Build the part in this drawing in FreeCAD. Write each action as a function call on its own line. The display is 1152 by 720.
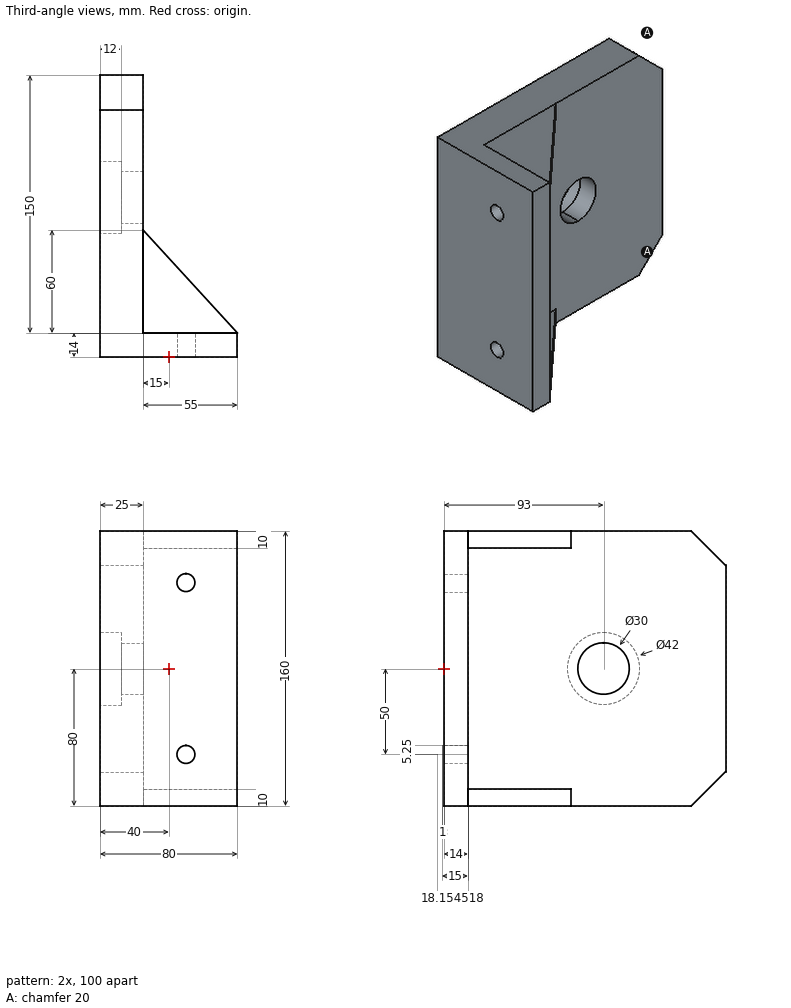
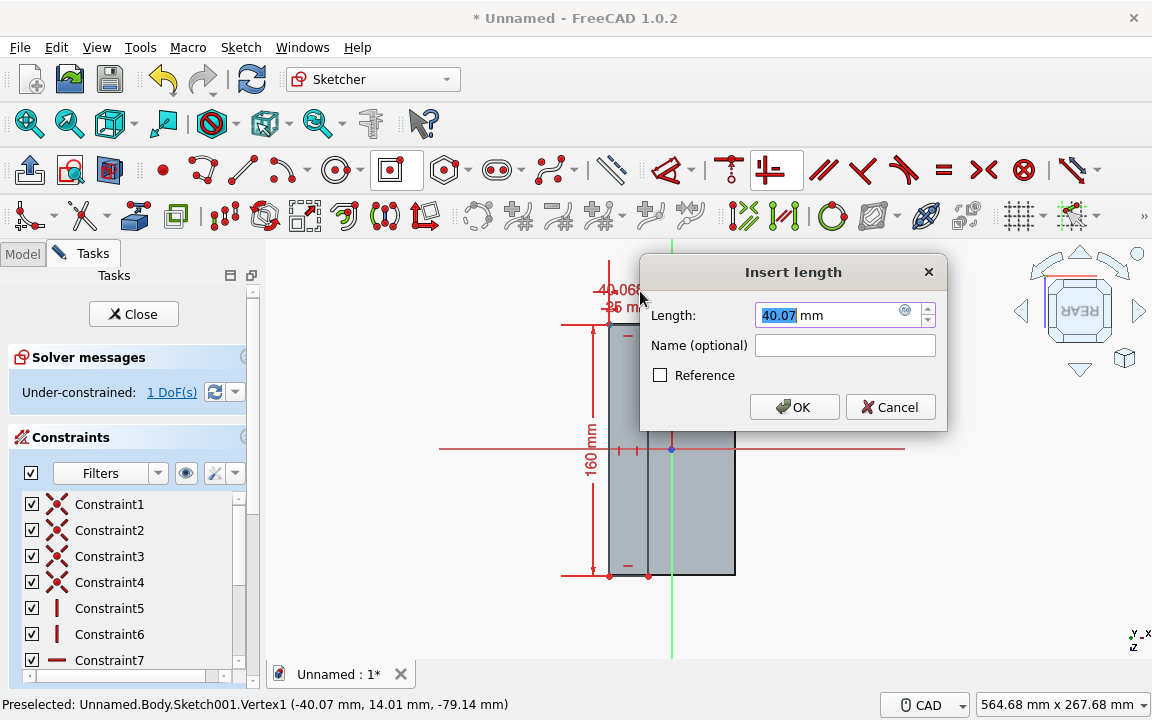
text(40)
key(Return)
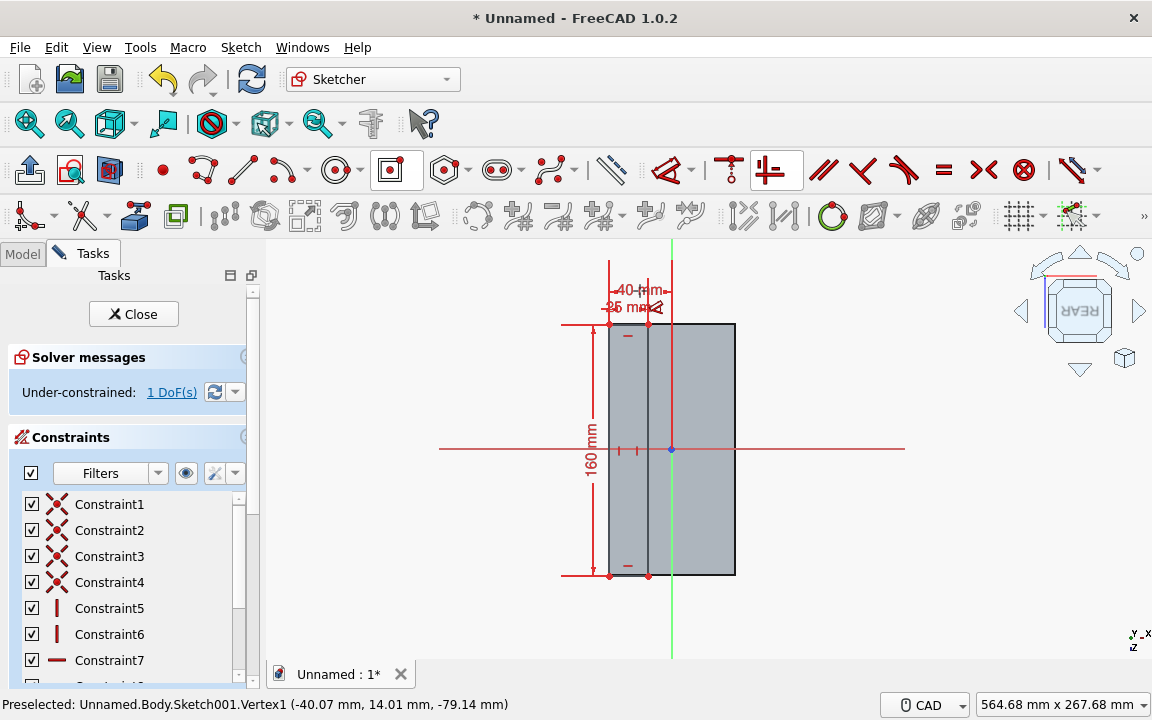
click(609, 325)
click(706, 387)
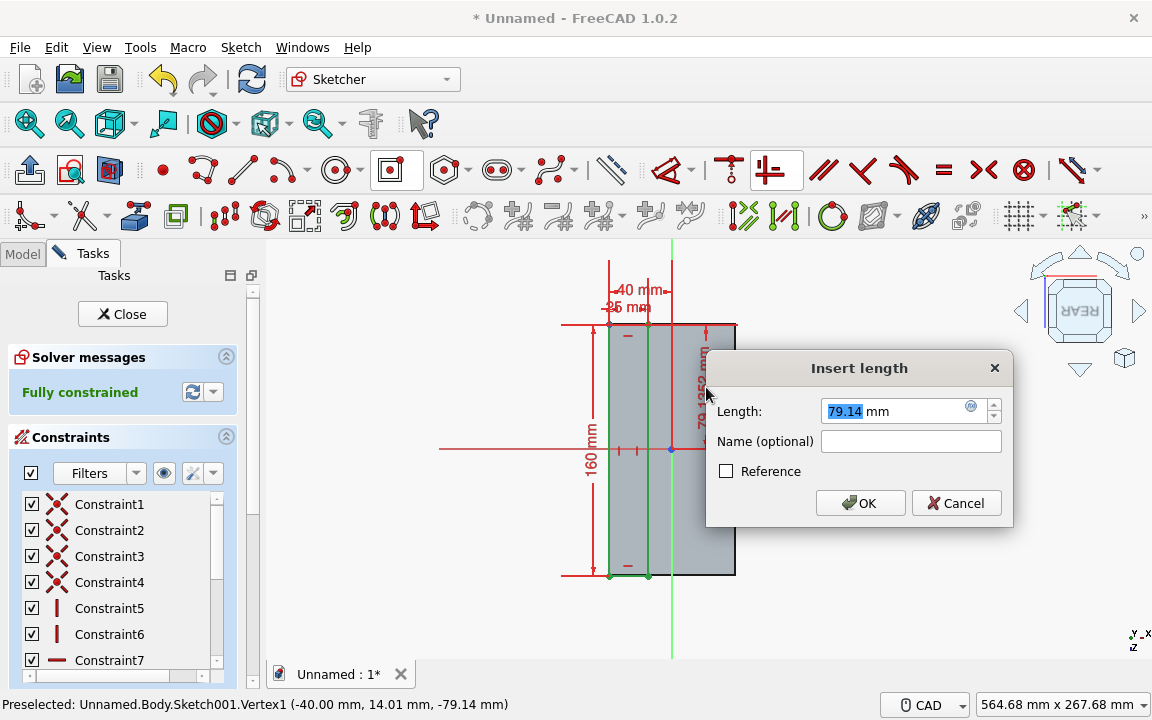
text(80)
key(Return)
key(Escape)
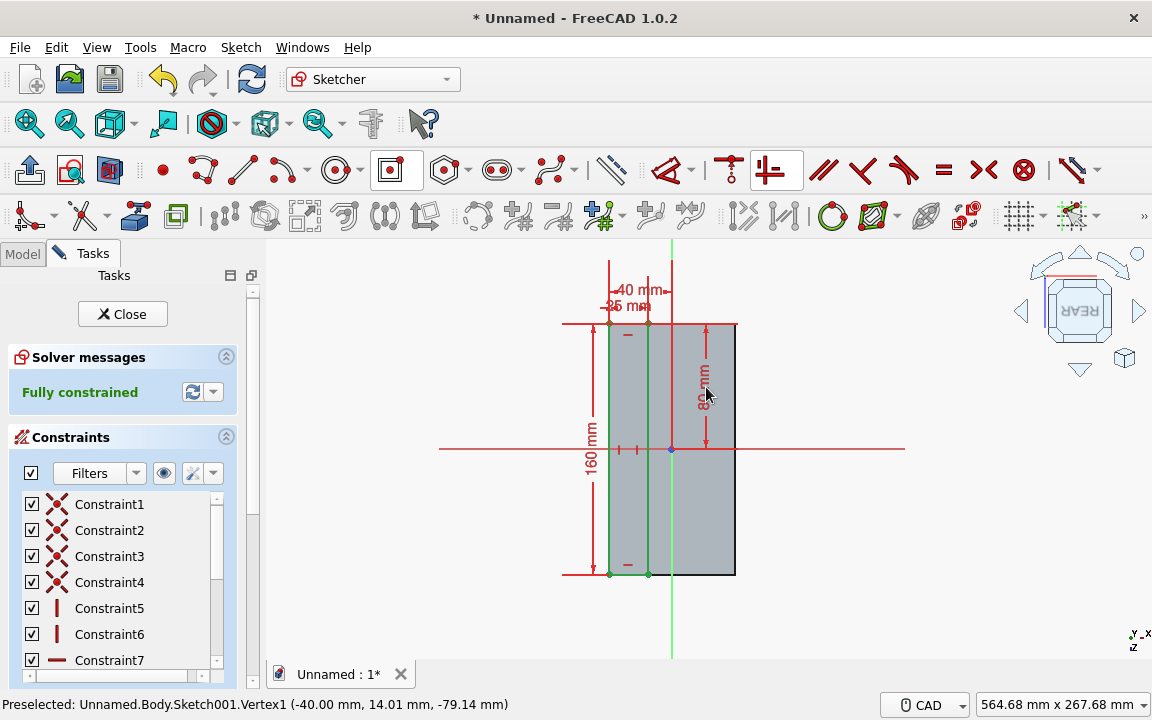
click(123, 314)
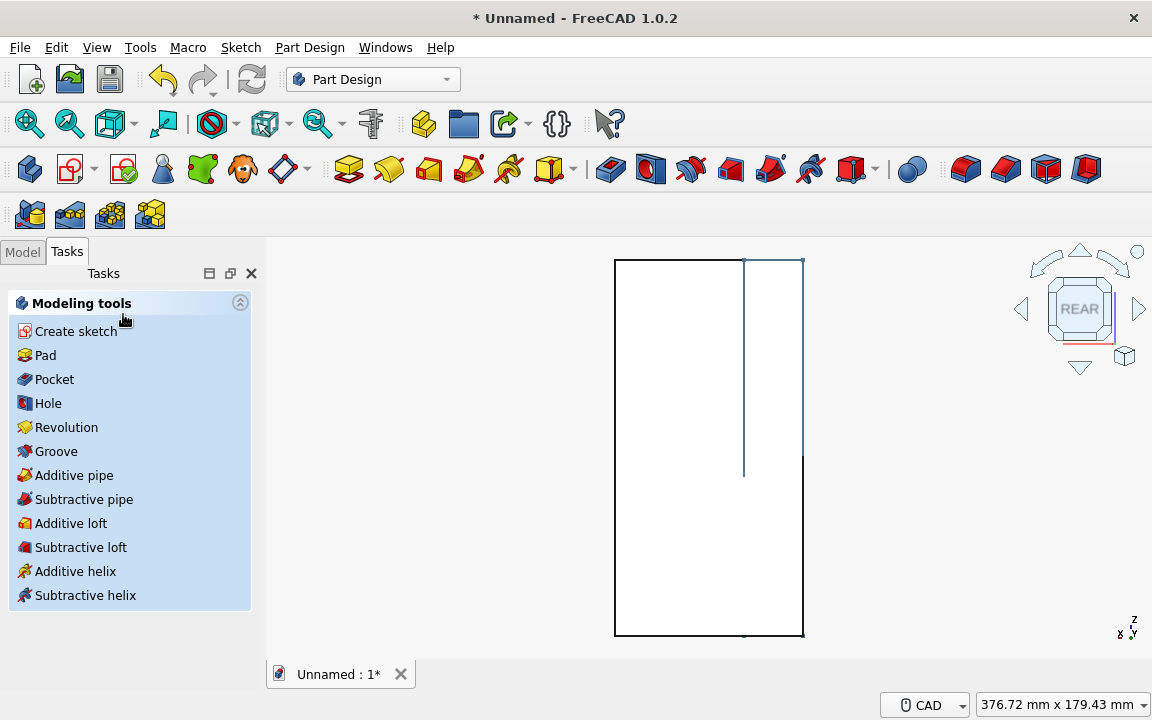
click(350, 170)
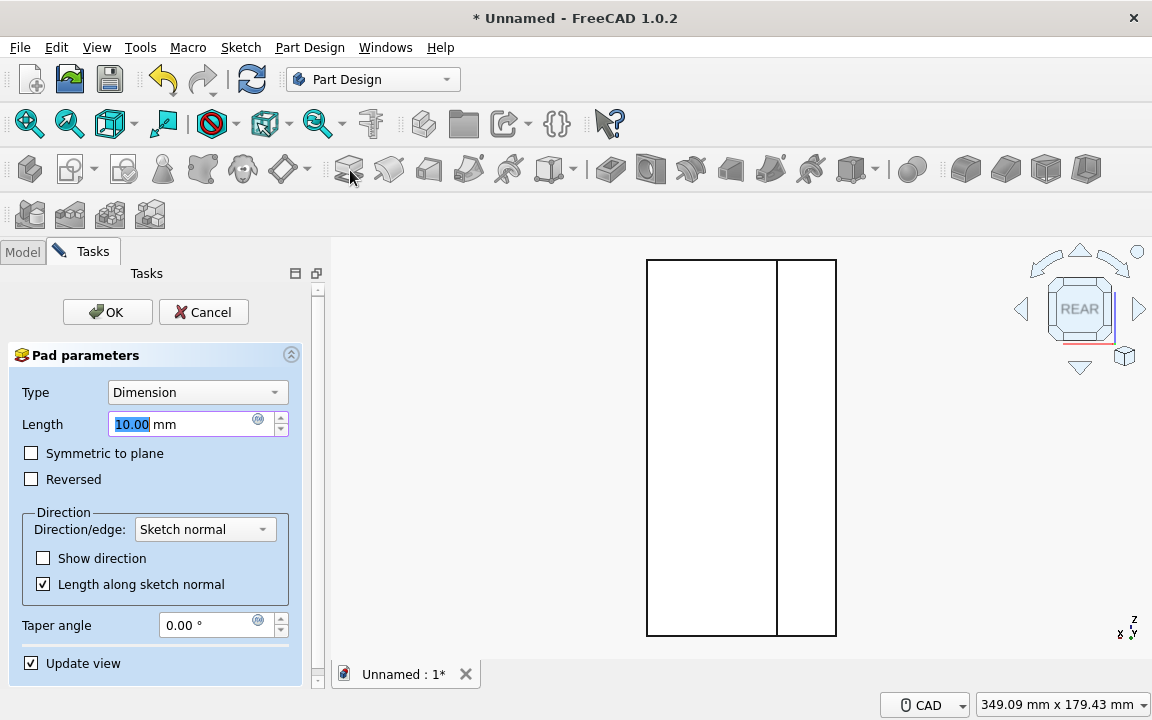
text(150)
key(Tab)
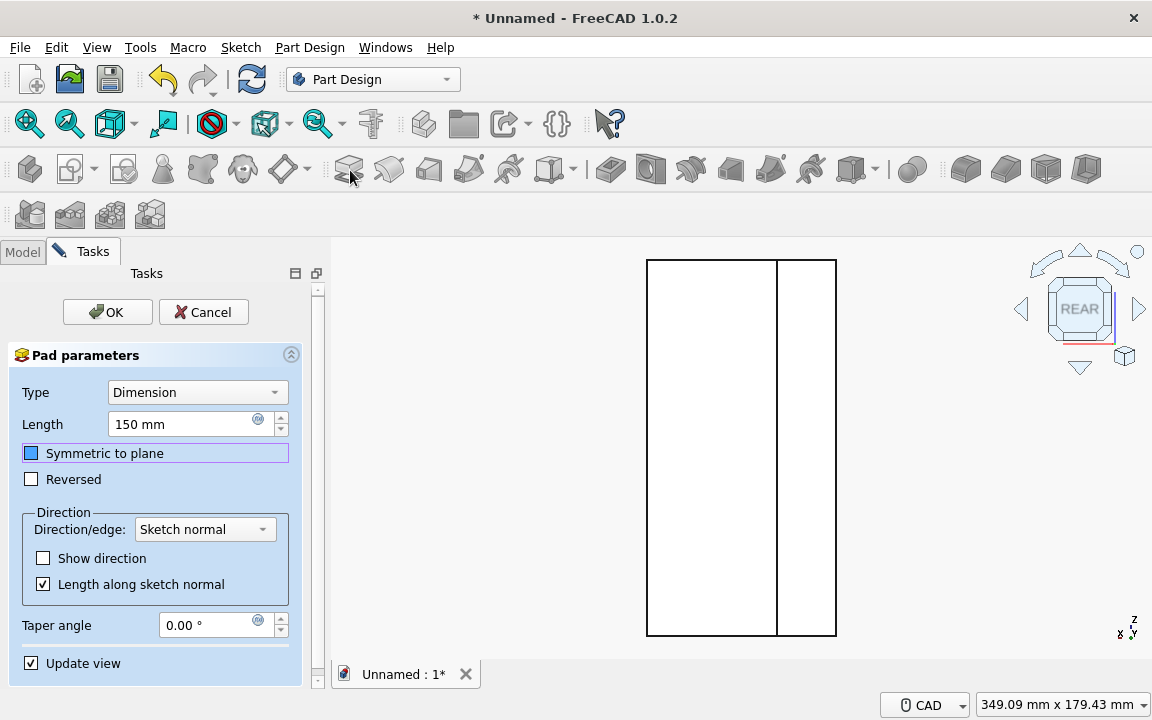
click(108, 312)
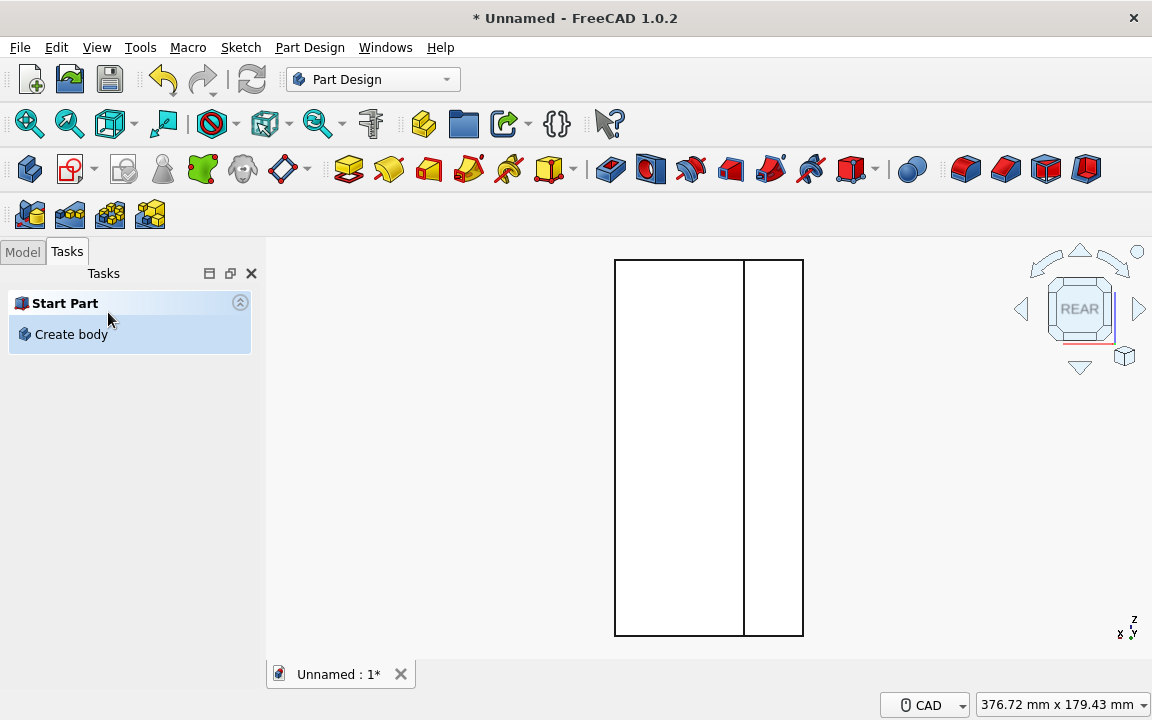
key(6)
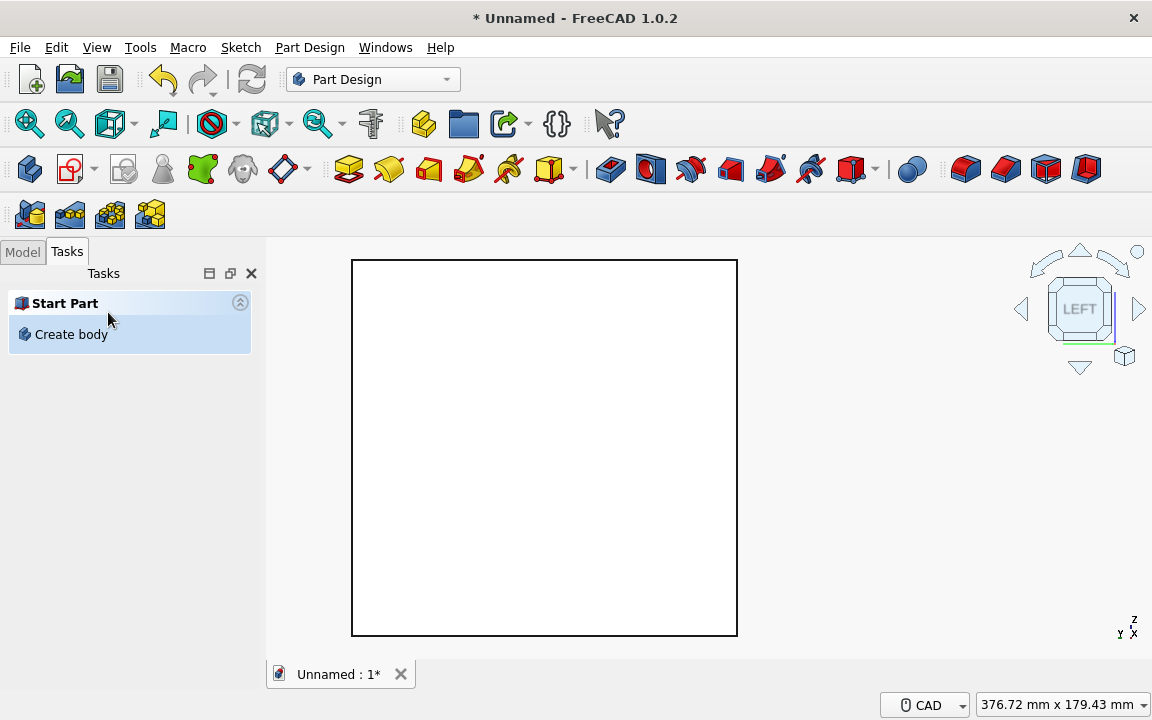
click(544, 447)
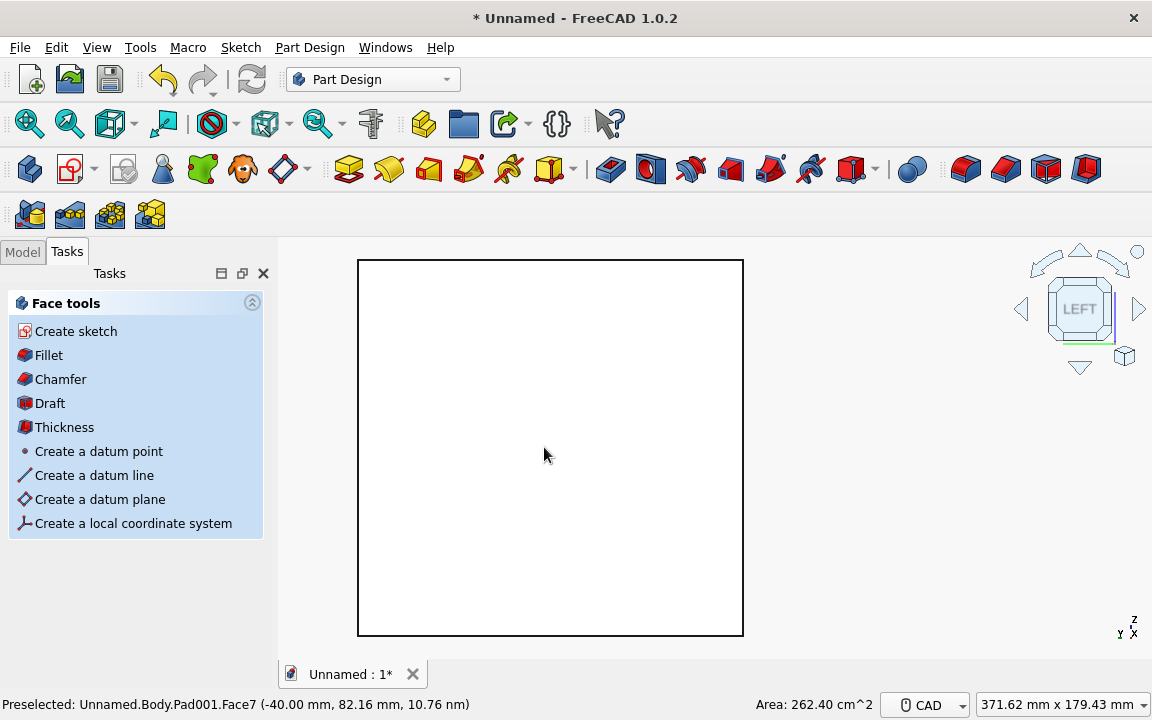
click(70, 170)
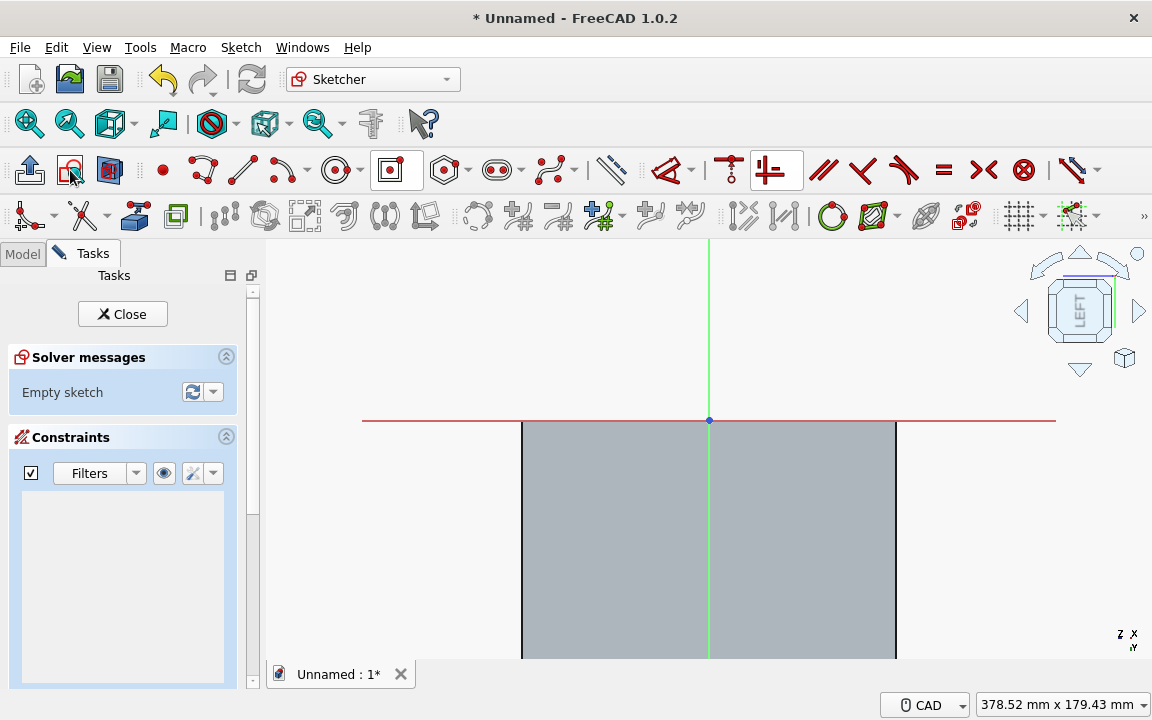
scroll(640, 449, down, 5)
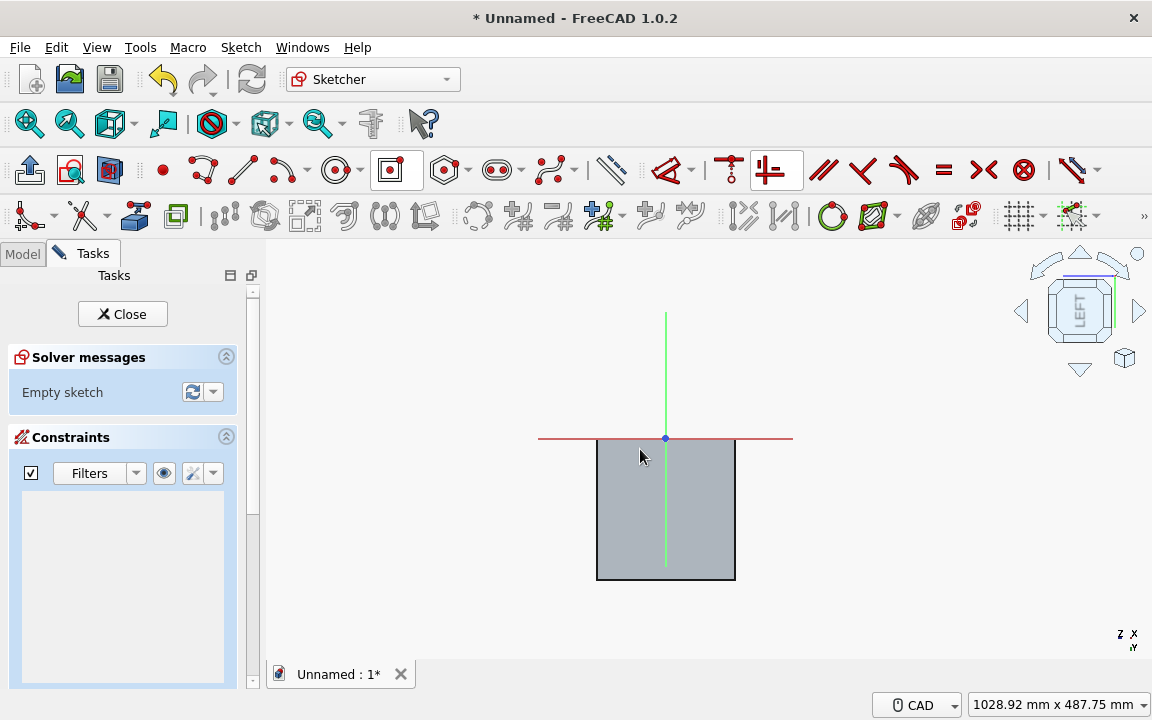
scroll(670, 530, up, 10)